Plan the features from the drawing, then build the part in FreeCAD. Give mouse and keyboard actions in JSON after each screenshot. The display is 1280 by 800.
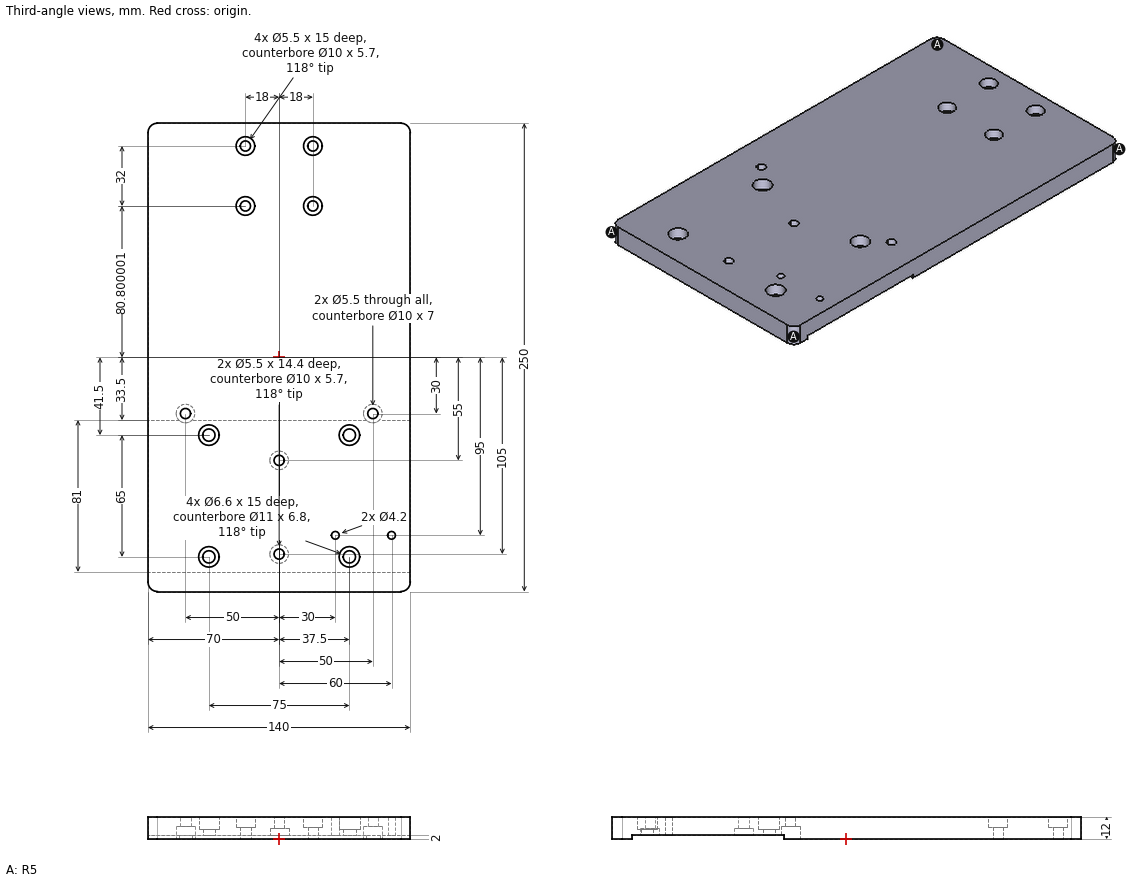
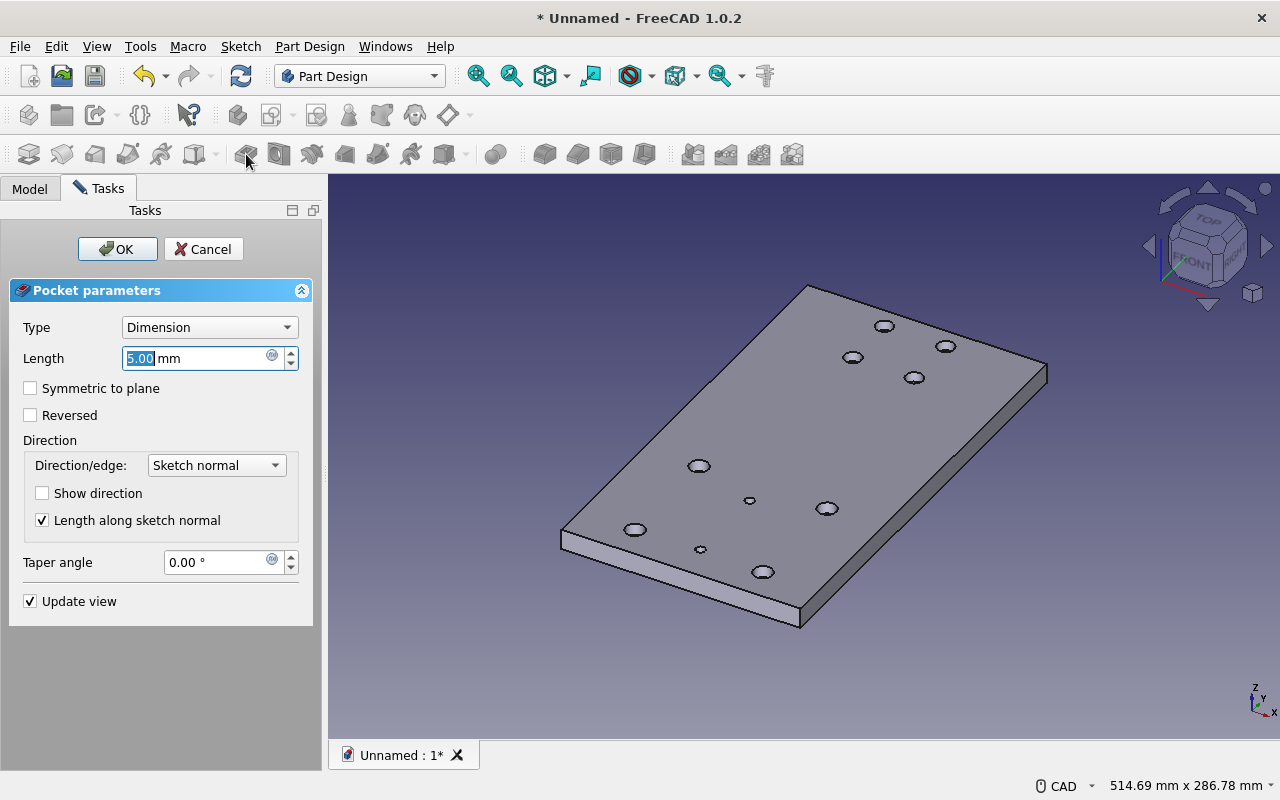
{"action": "type", "text": "2"}
{"action": "key", "text": "Tab"}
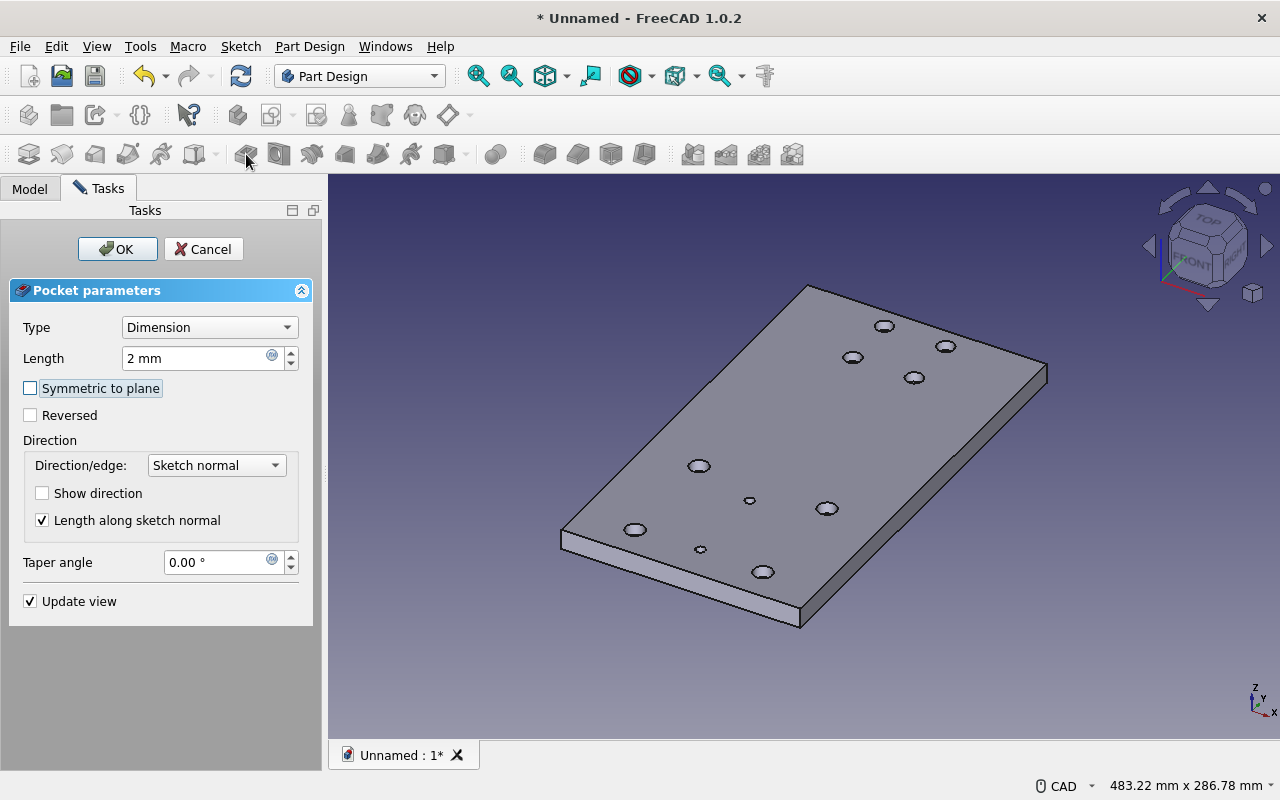
{"action": "left_click", "coordinate": [31, 415]}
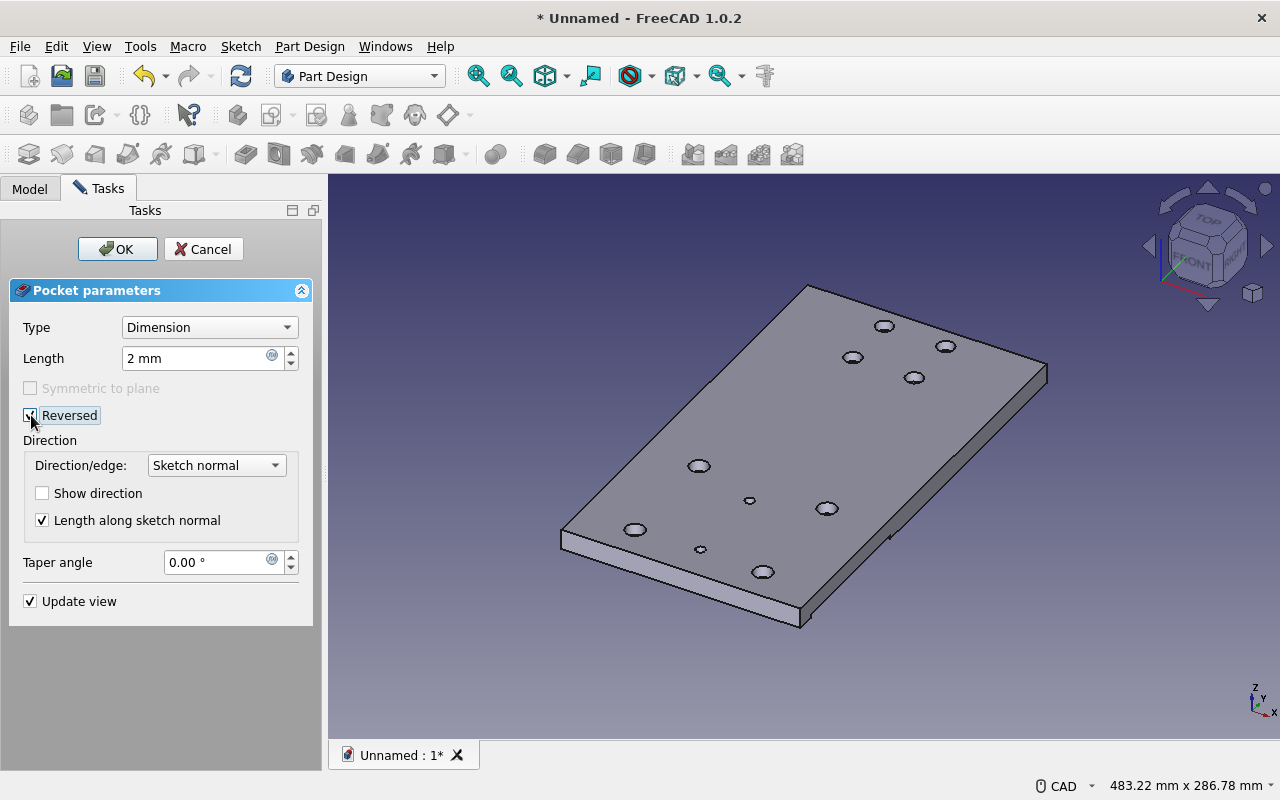
{"action": "left_click", "coordinate": [118, 249]}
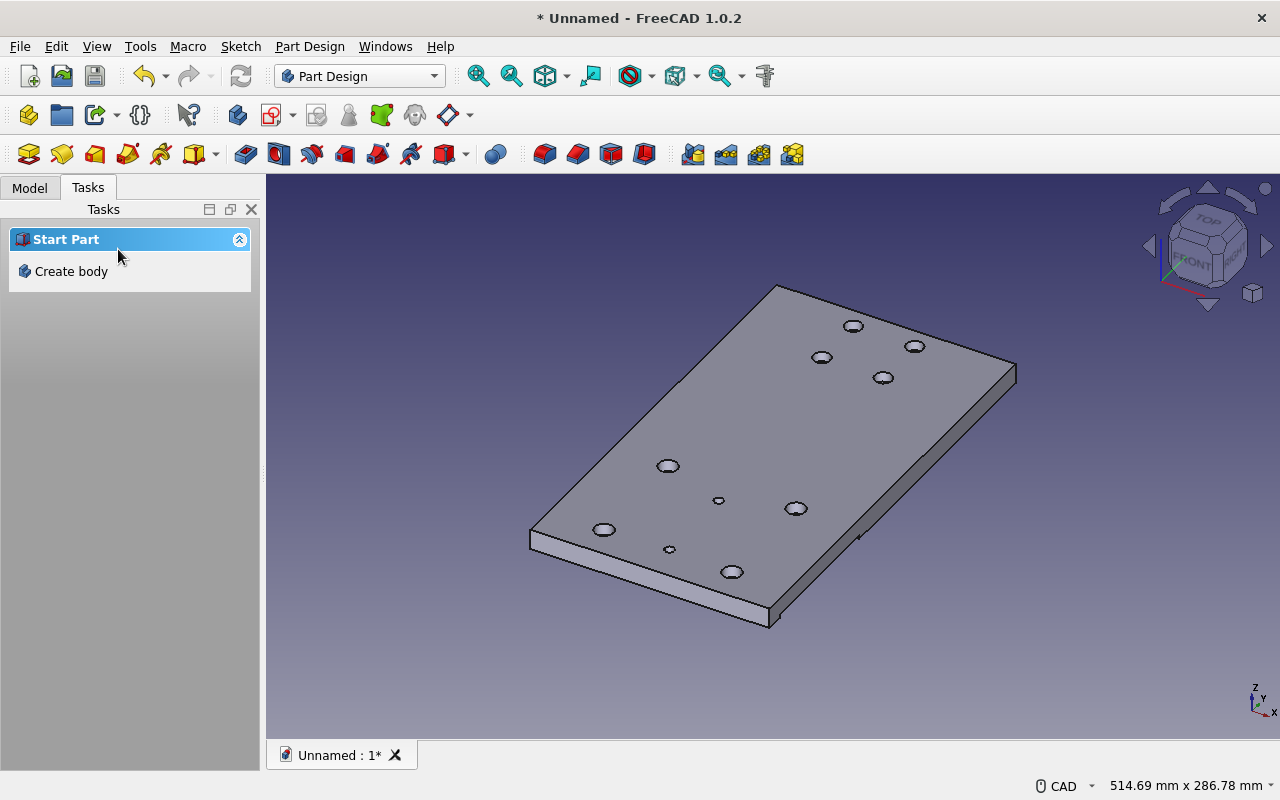
{"action": "left_click", "coordinate": [270, 116]}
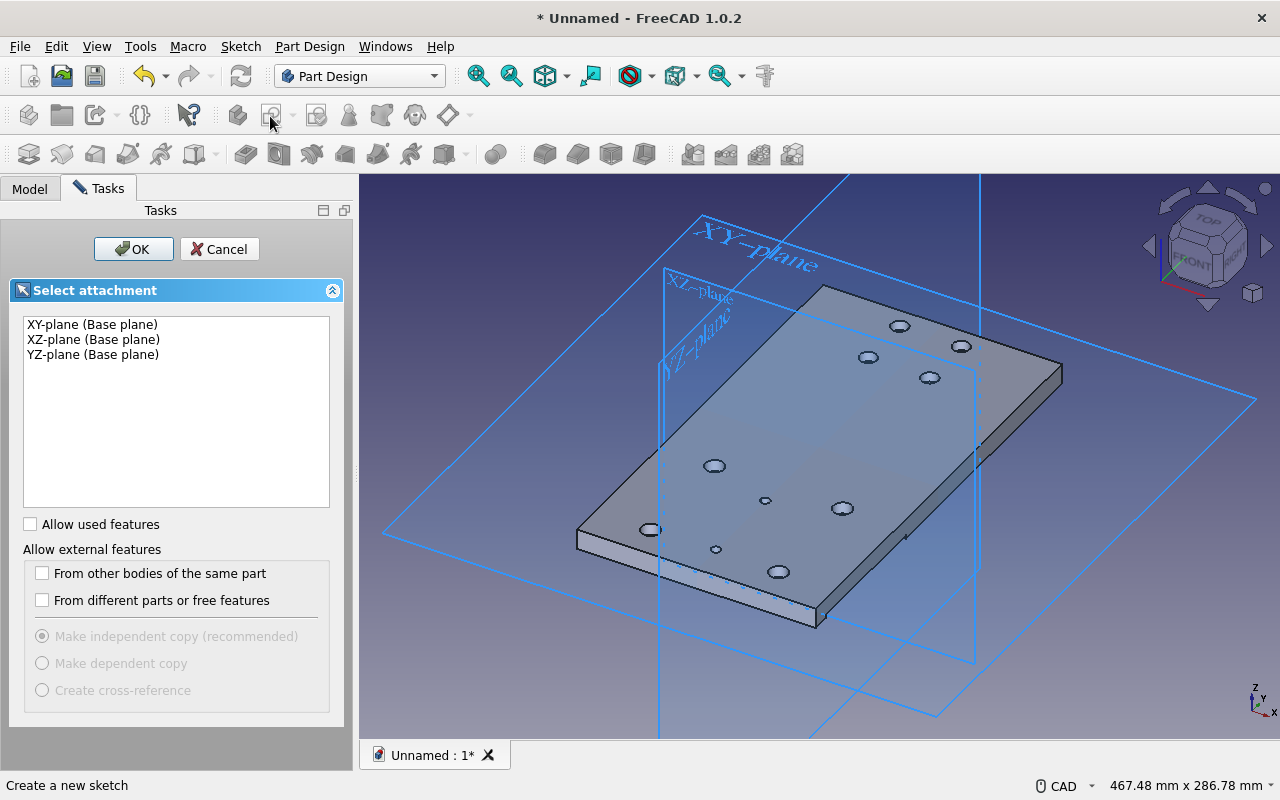
{"action": "left_click", "coordinate": [84, 324]}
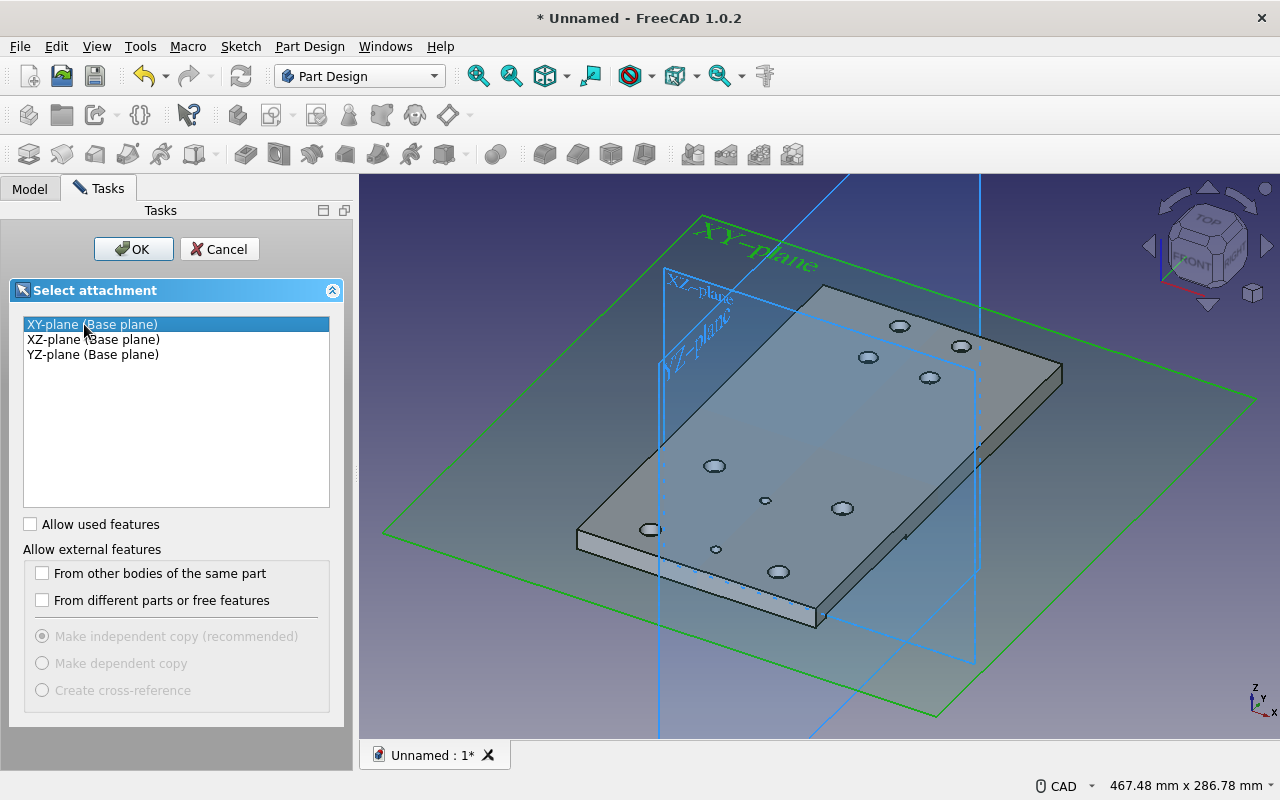
{"action": "left_click", "coordinate": [134, 249]}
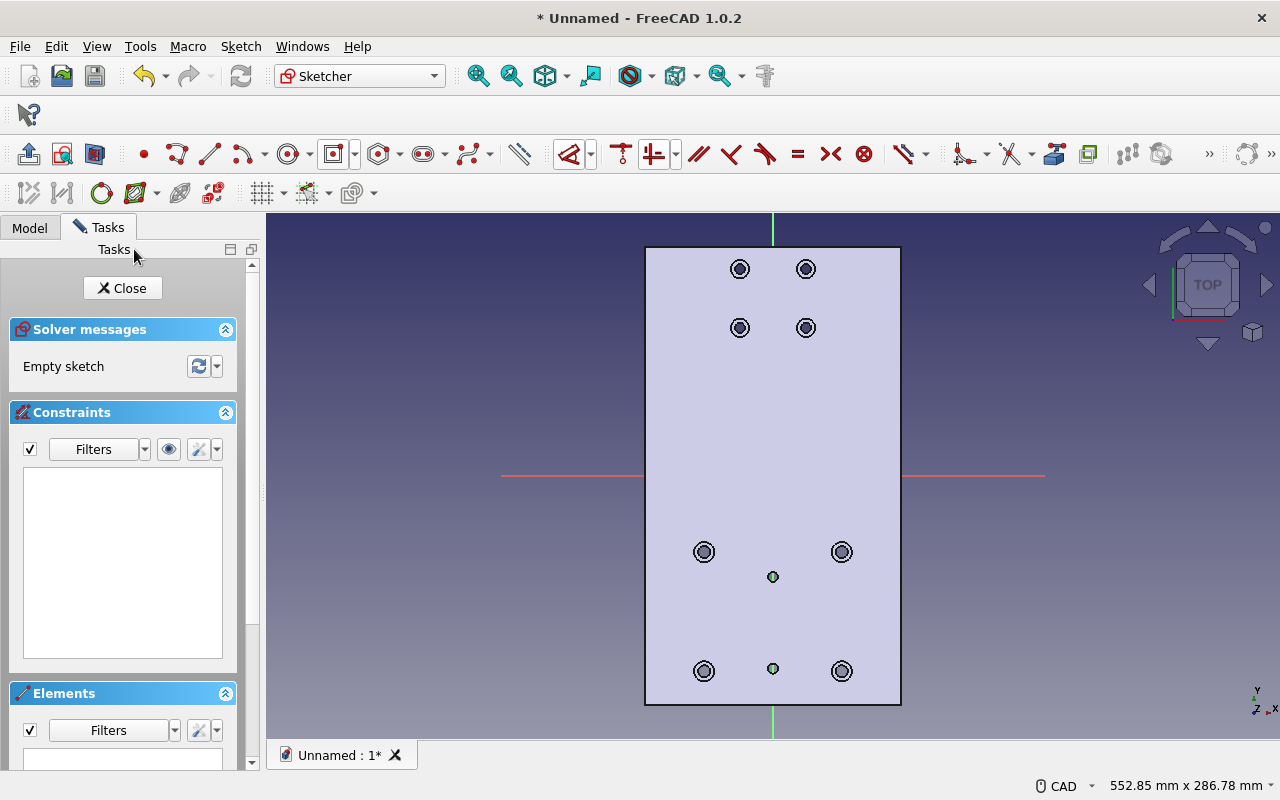
{"action": "left_click", "coordinate": [95, 154]}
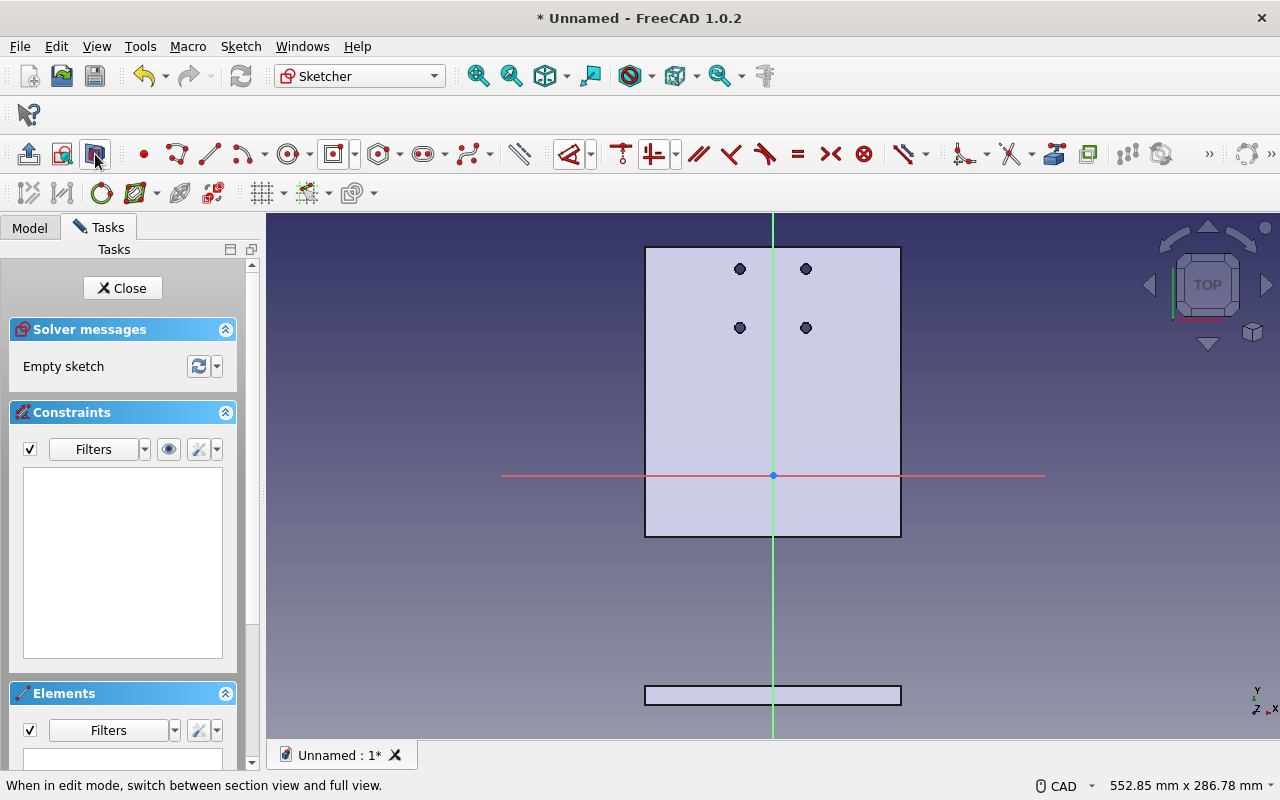
{"action": "scroll", "coordinate": [813, 524], "scroll_direction": "up", "scroll_amount": 5}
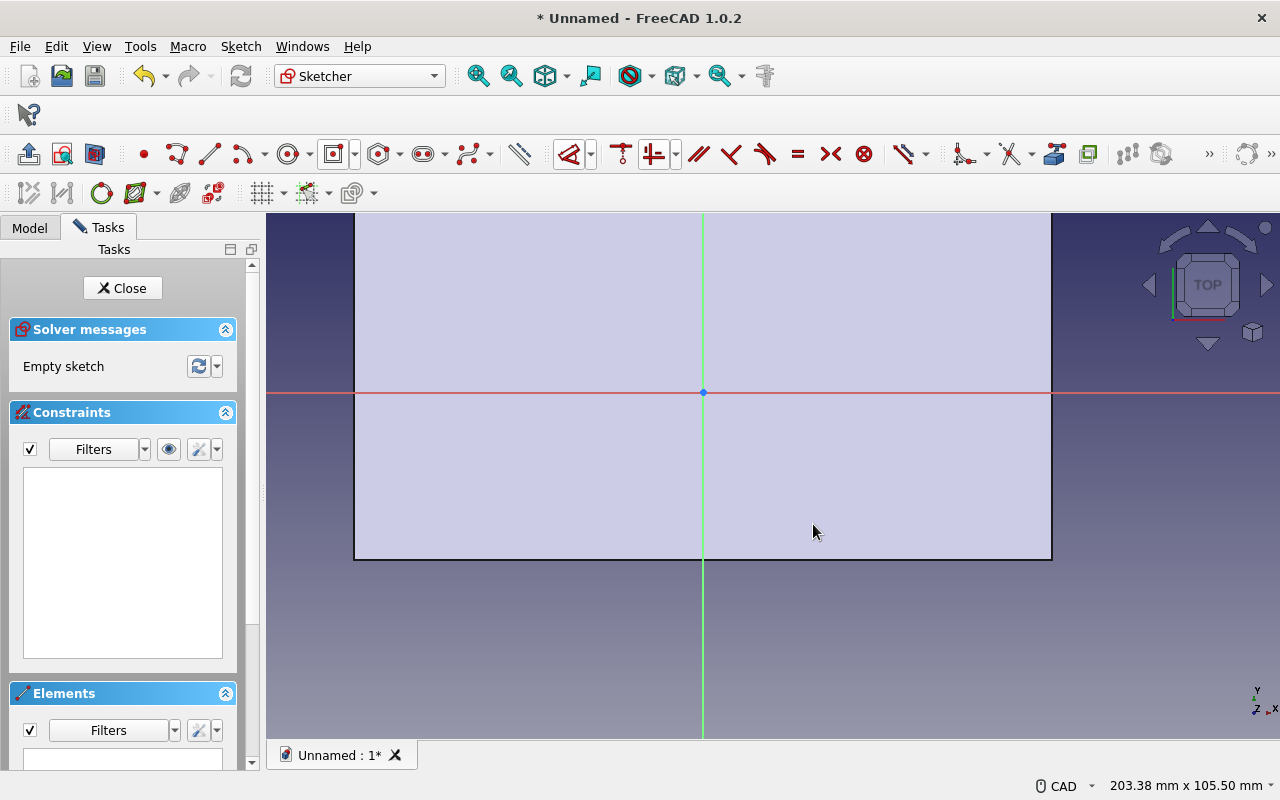
{"action": "key", "text": "g c"}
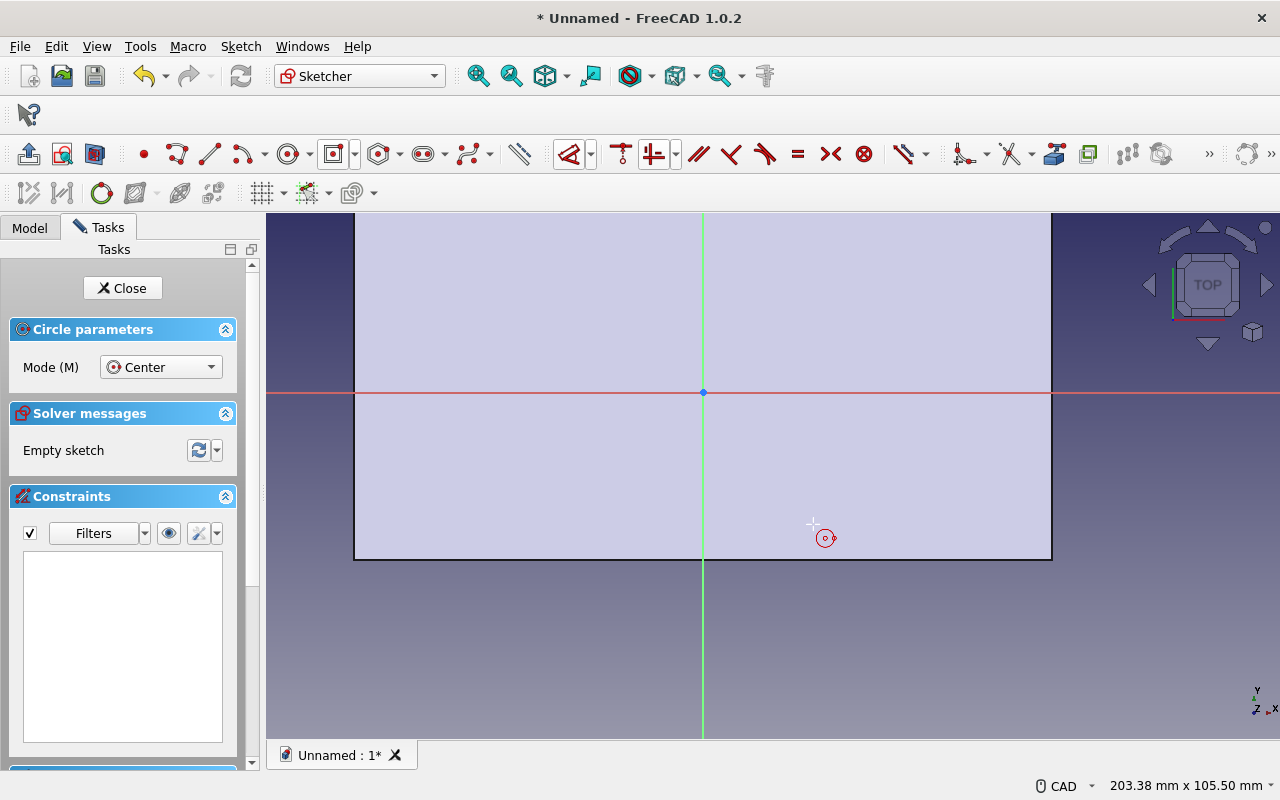
{"action": "scroll", "coordinate": [953, 542], "scroll_direction": "up", "scroll_amount": 3}